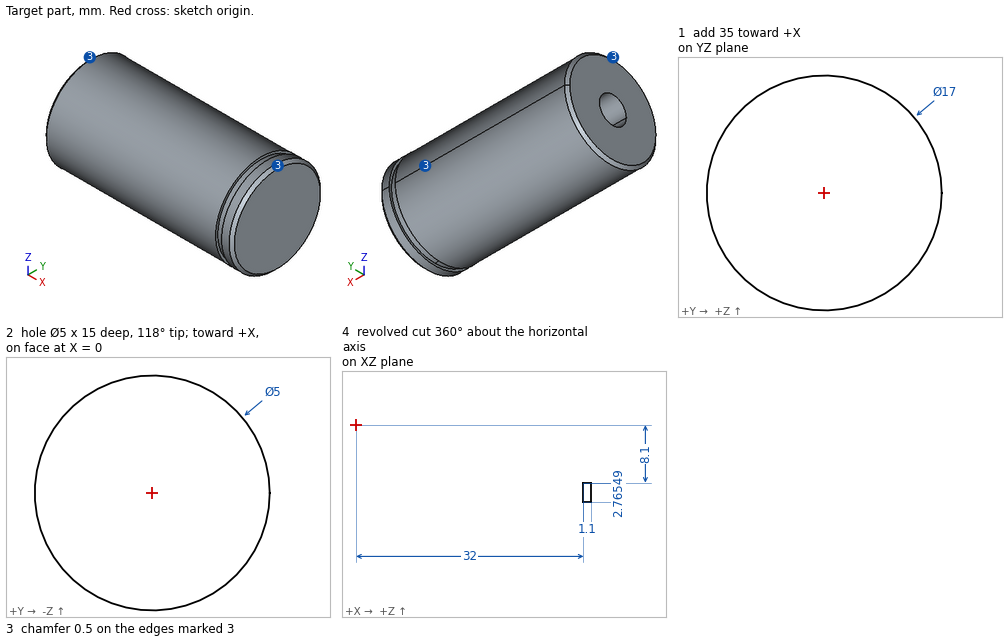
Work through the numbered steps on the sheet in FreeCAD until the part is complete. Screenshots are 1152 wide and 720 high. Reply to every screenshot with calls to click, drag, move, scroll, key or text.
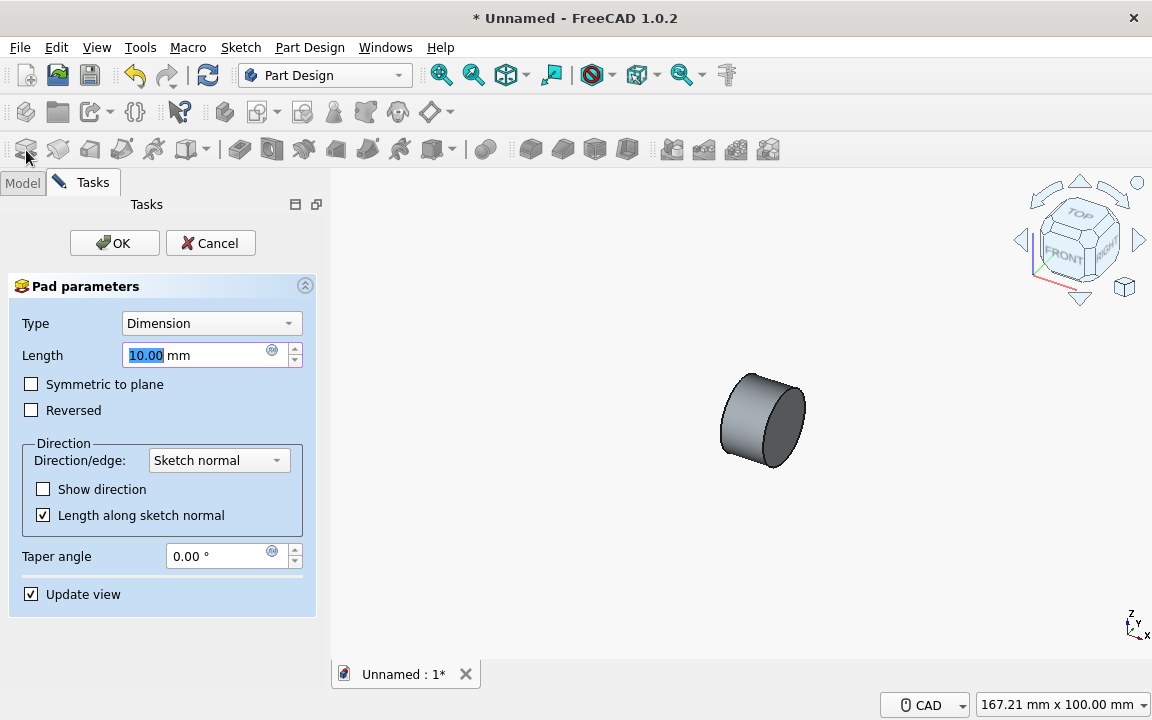
text(35)
key(Tab)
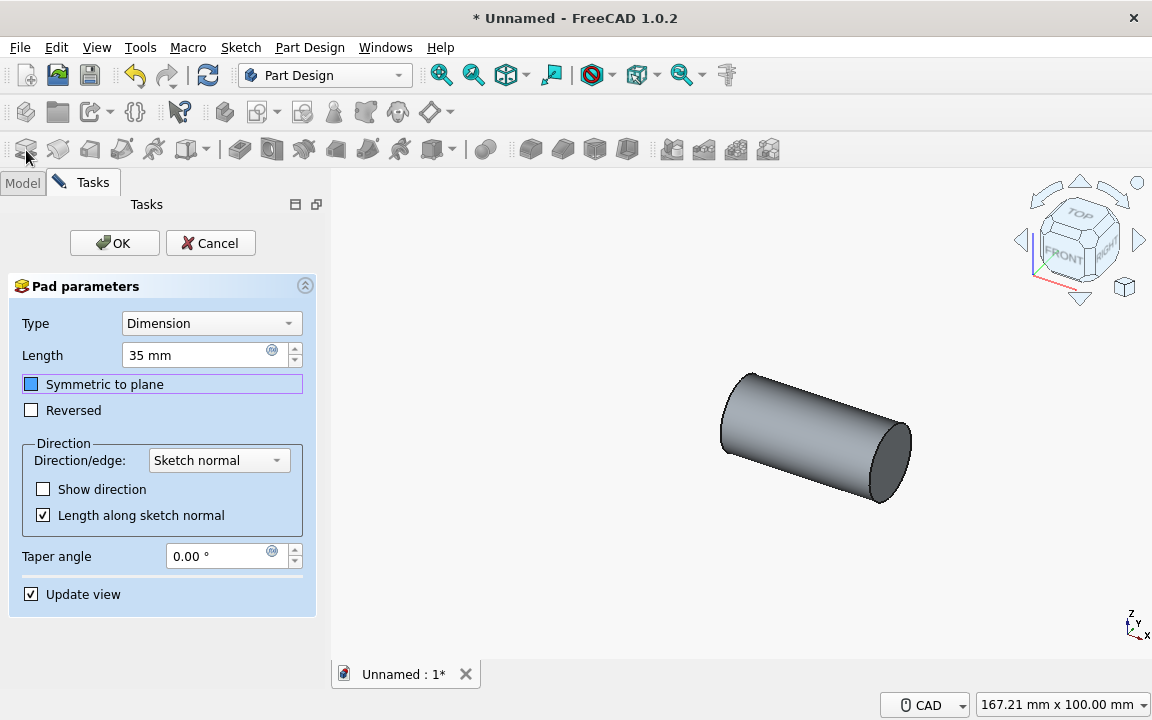
click(115, 243)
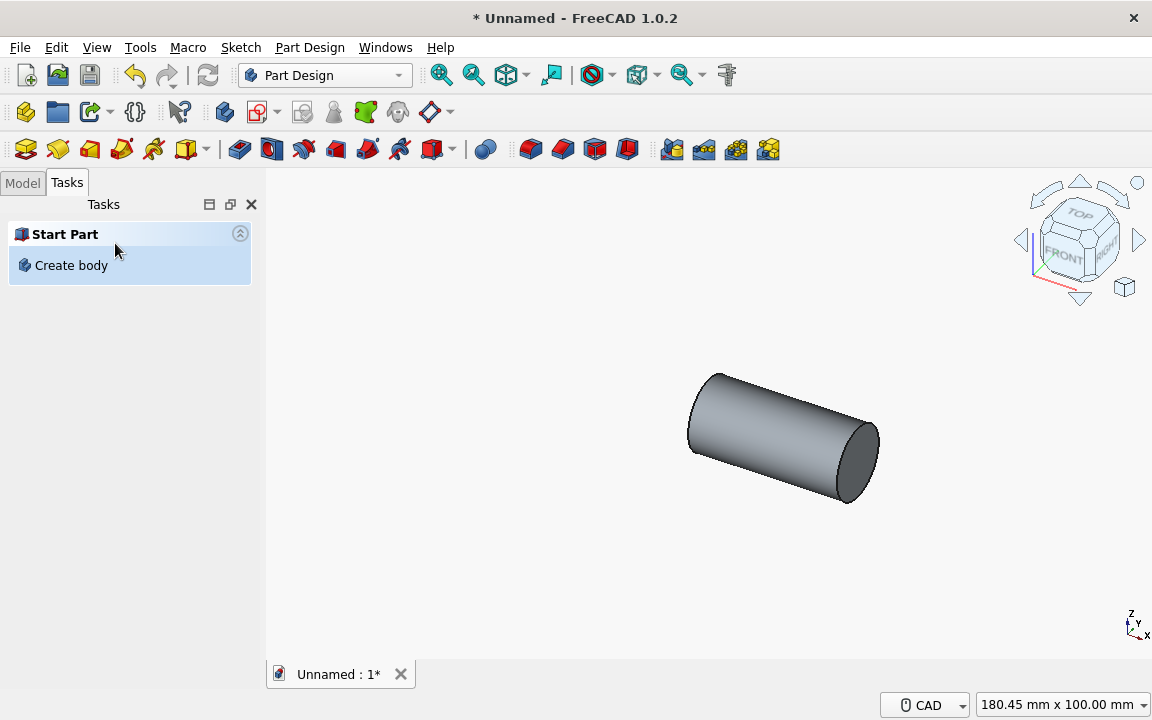
click(442, 76)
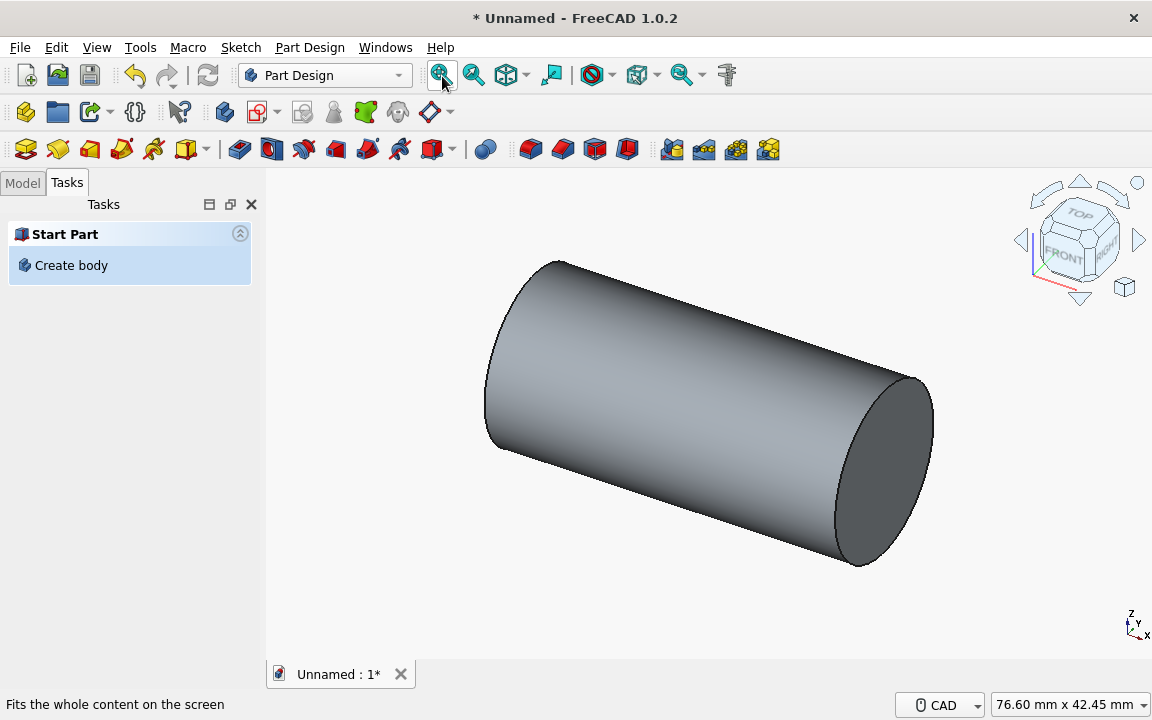
key(6)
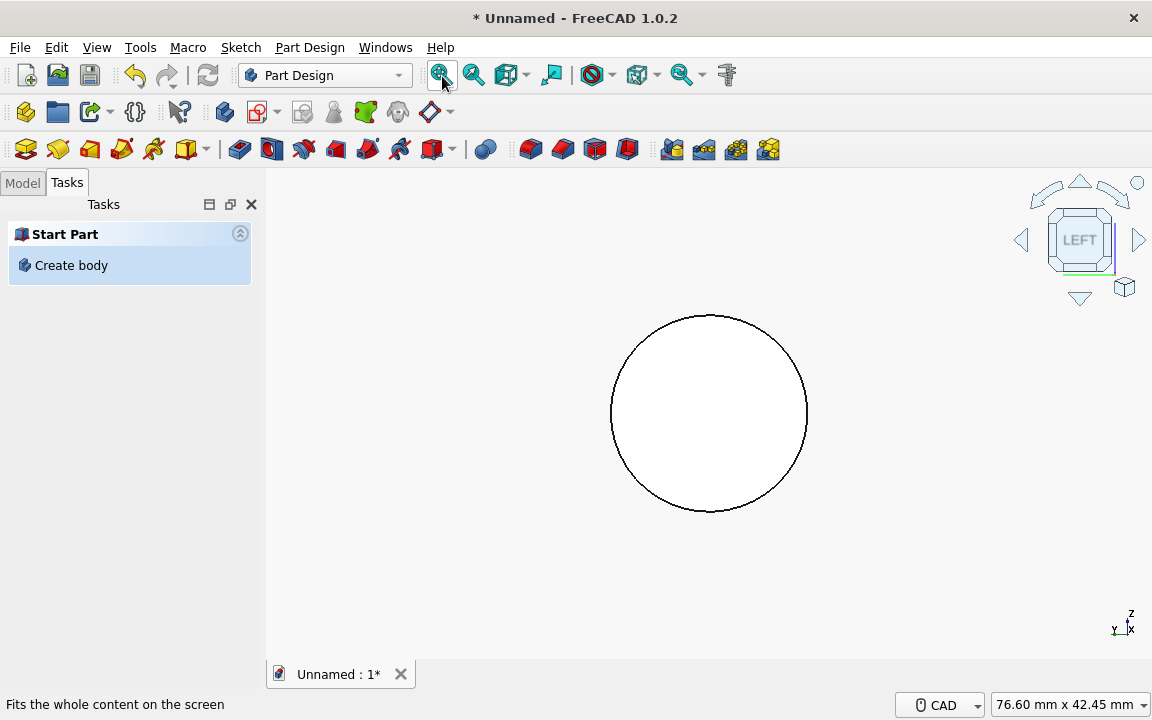
click(442, 76)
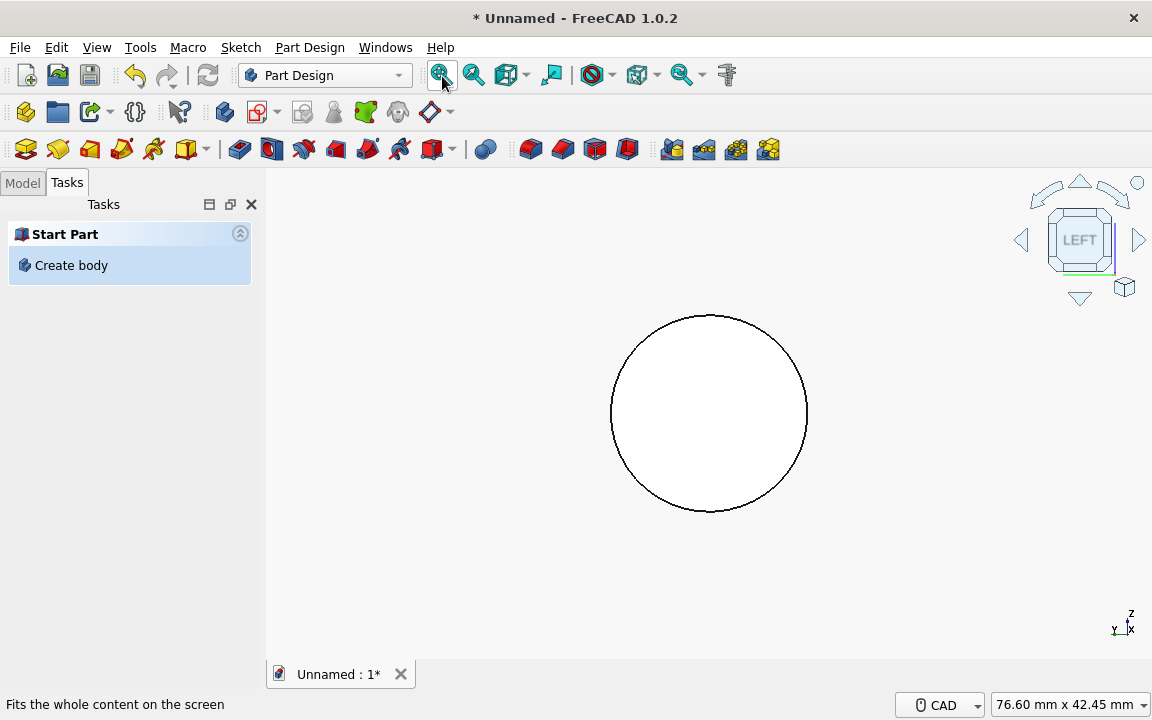
click(709, 412)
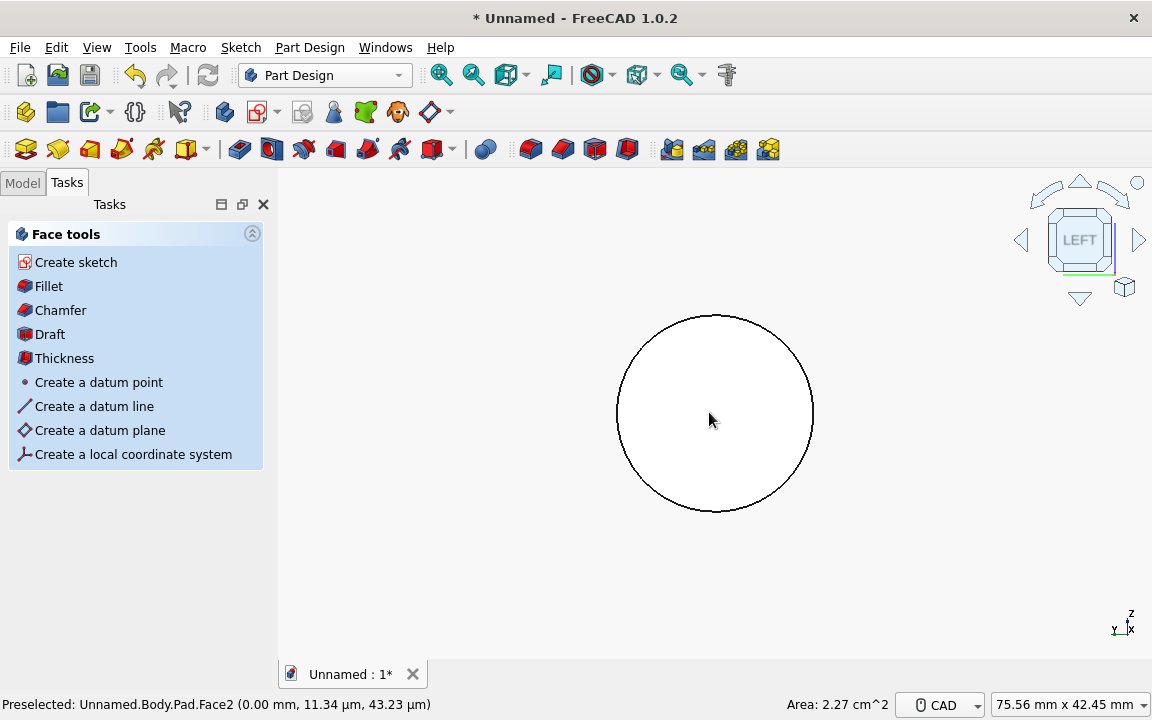
click(258, 112)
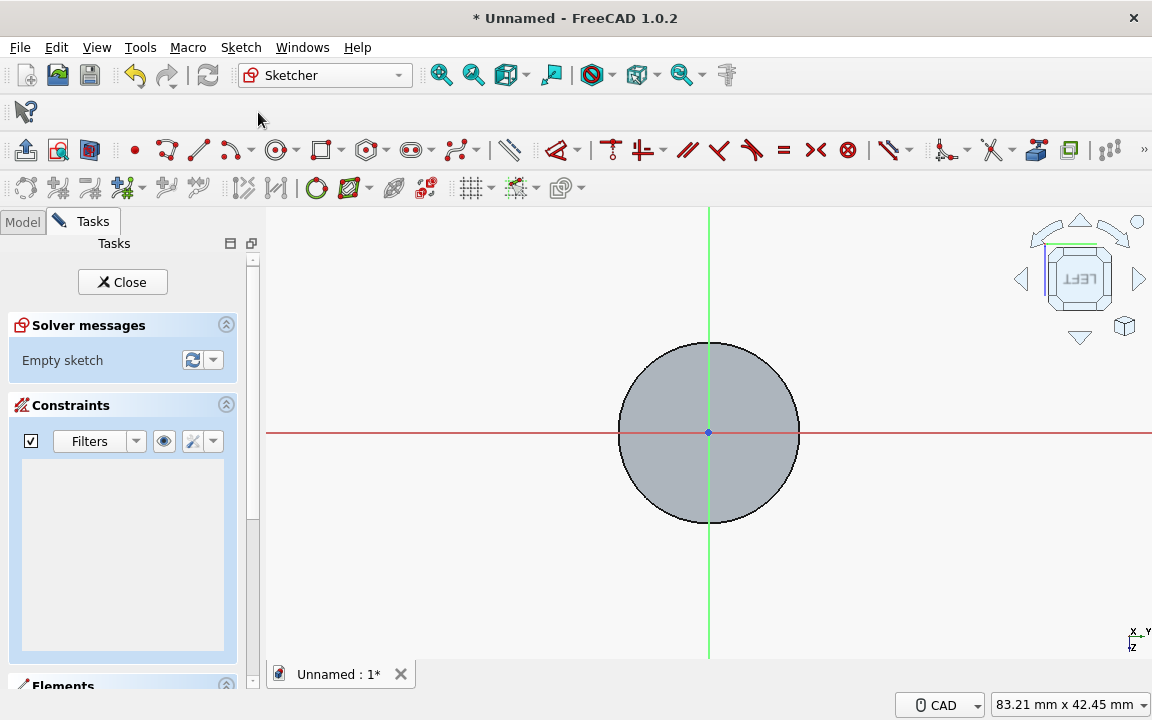
scroll(726, 433, up, 8)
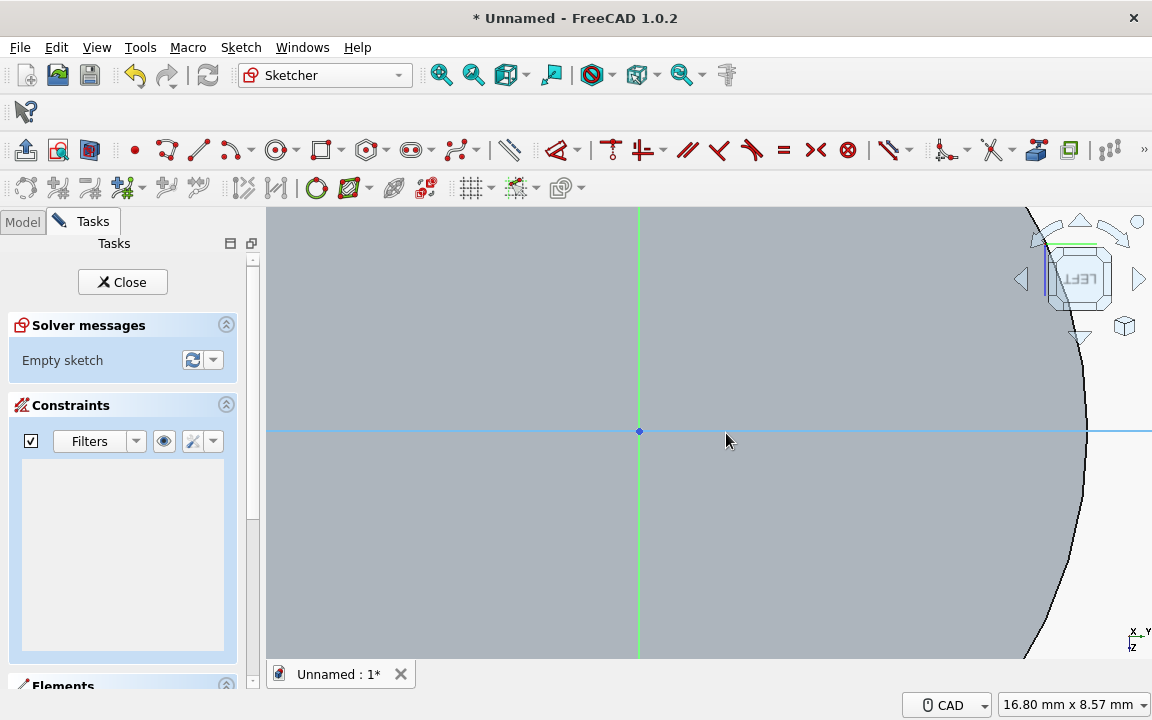
click(276, 150)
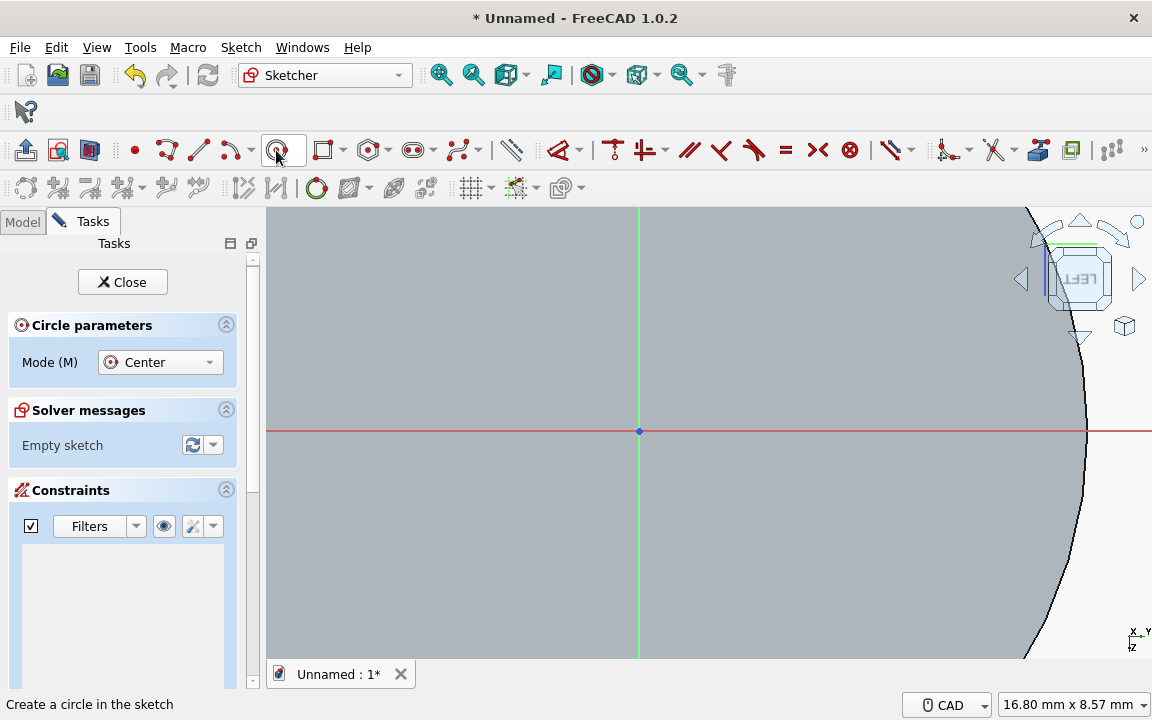
click(639, 431)
click(732, 338)
key(Escape)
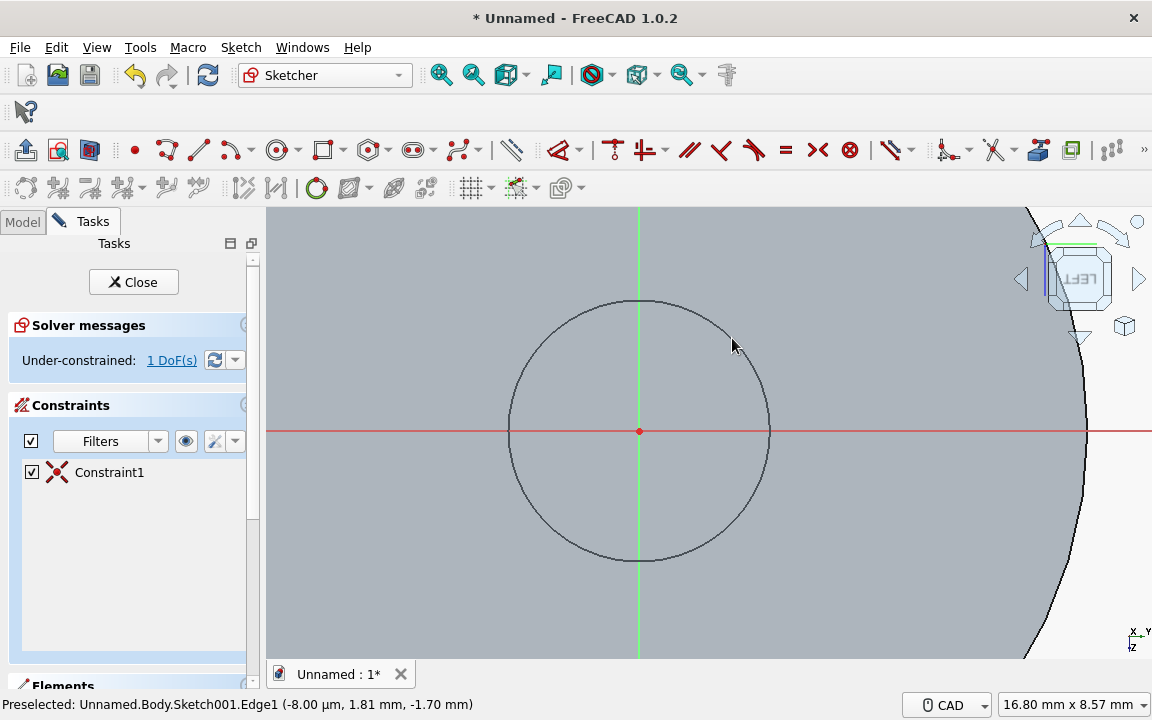
click(558, 150)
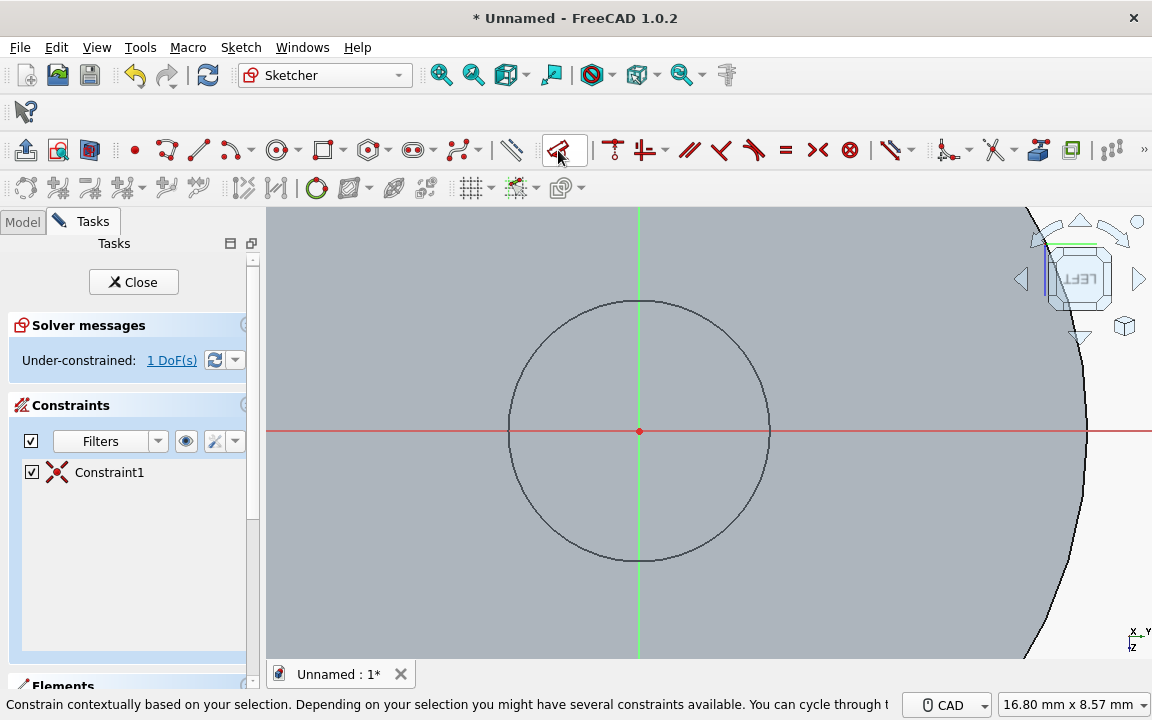
click(731, 338)
click(753, 315)